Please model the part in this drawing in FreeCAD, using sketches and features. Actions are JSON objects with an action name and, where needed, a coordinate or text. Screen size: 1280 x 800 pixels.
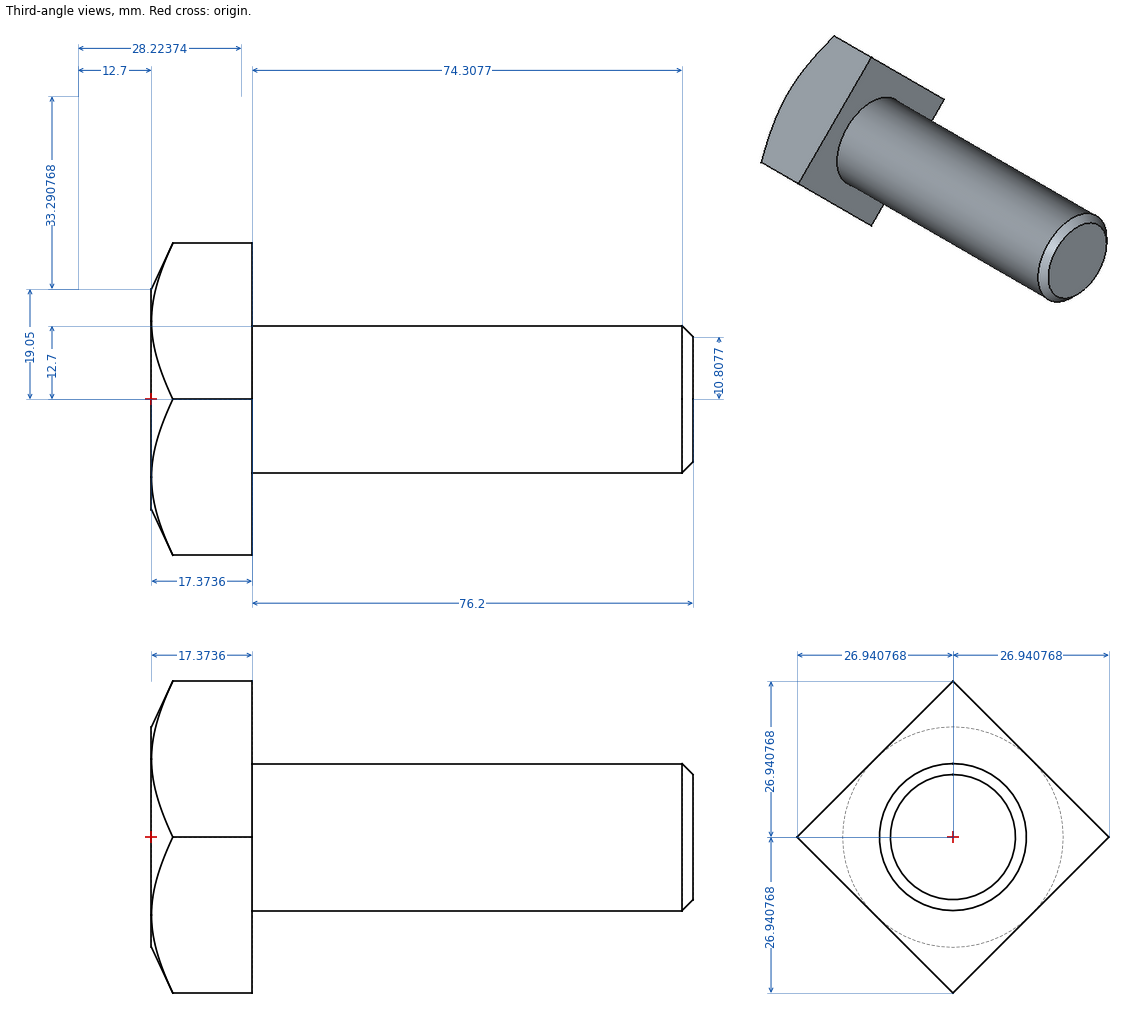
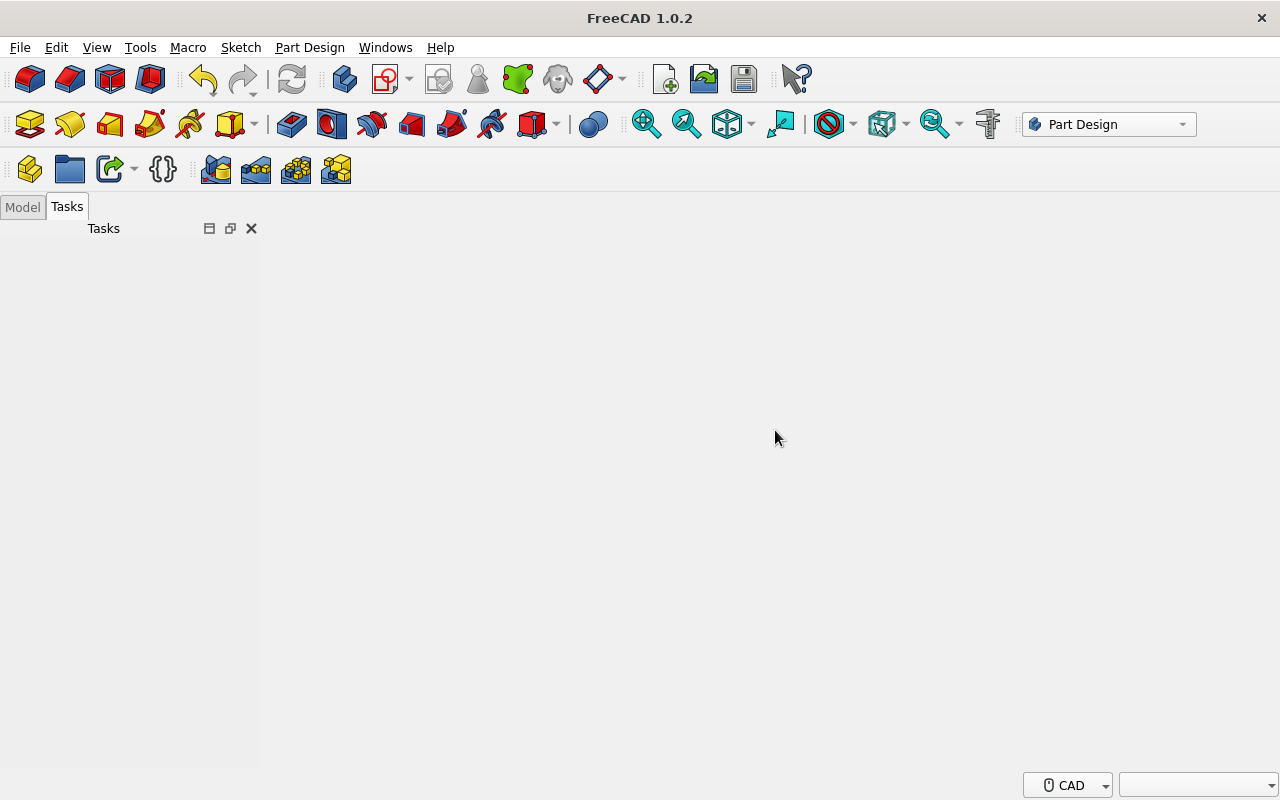
{"action": "left_click", "coordinate": [664, 80]}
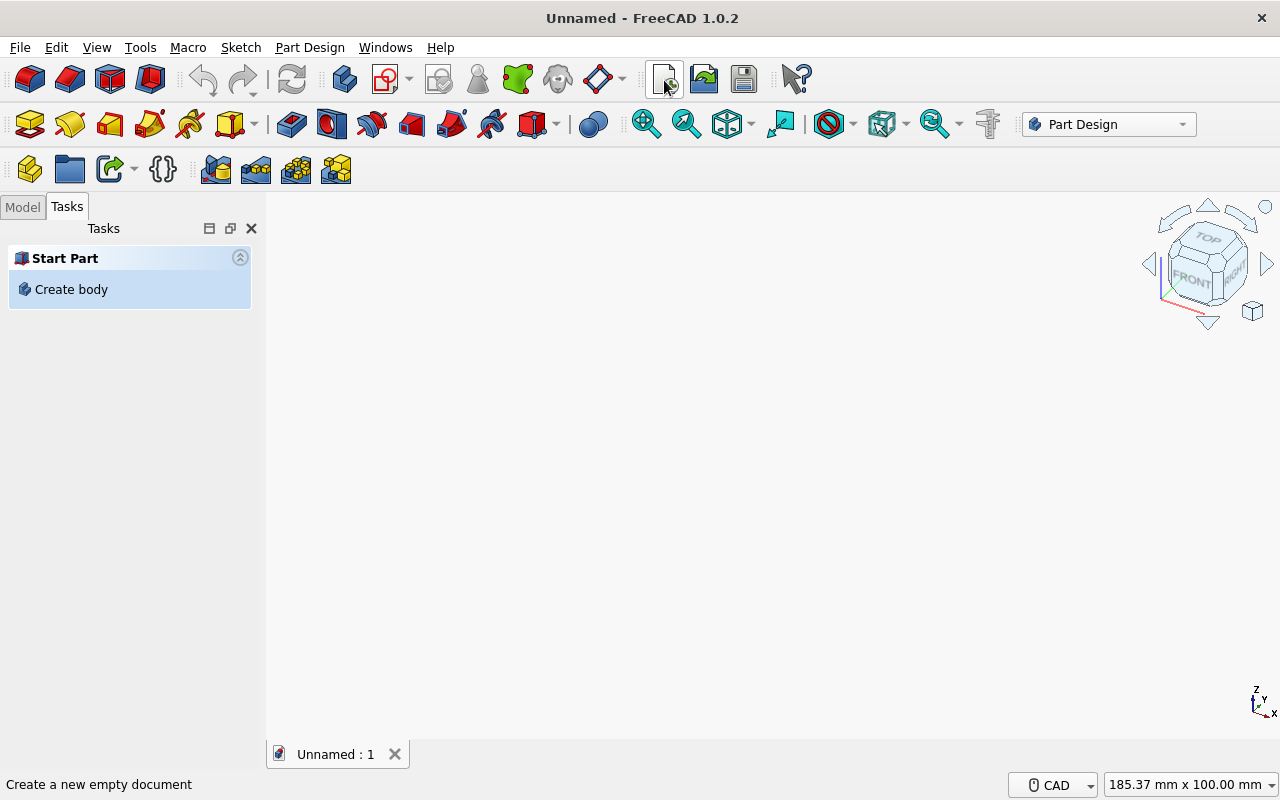
{"action": "left_click", "coordinate": [386, 80]}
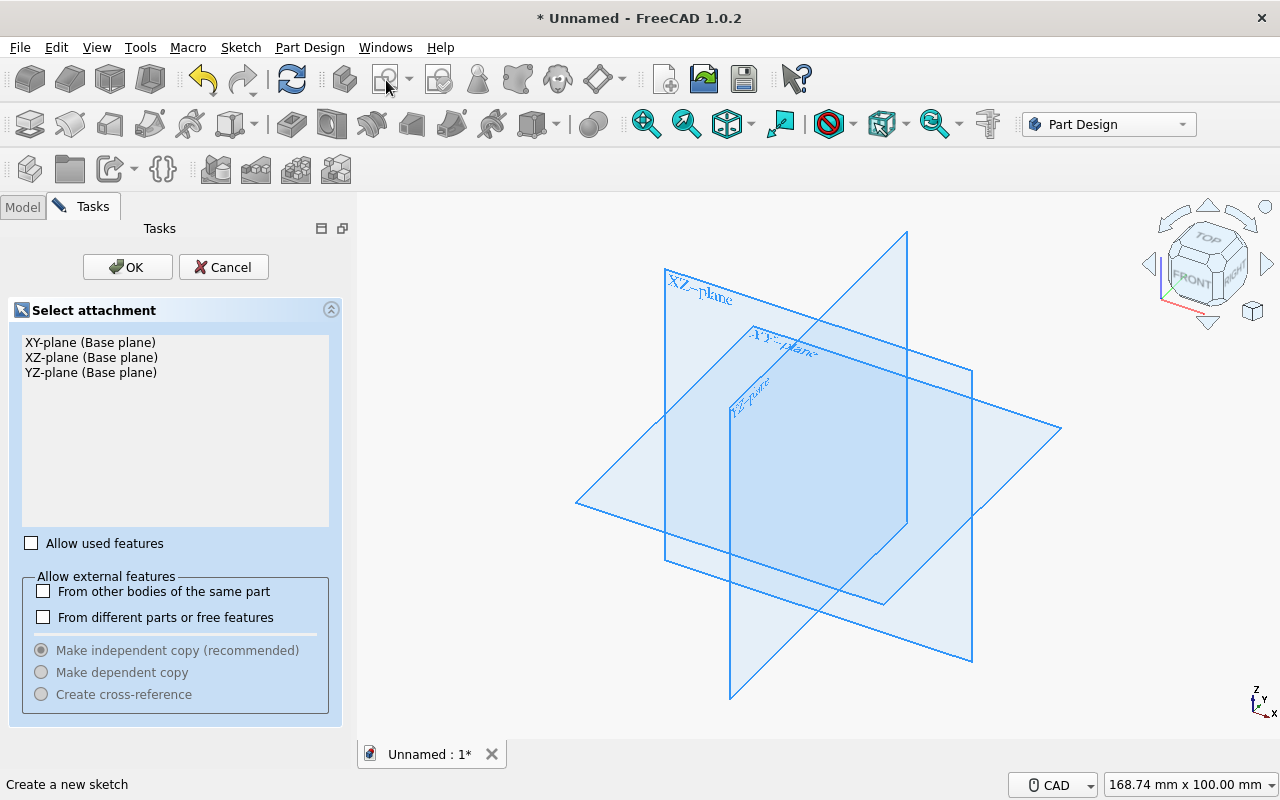
{"action": "left_click", "coordinate": [82, 372]}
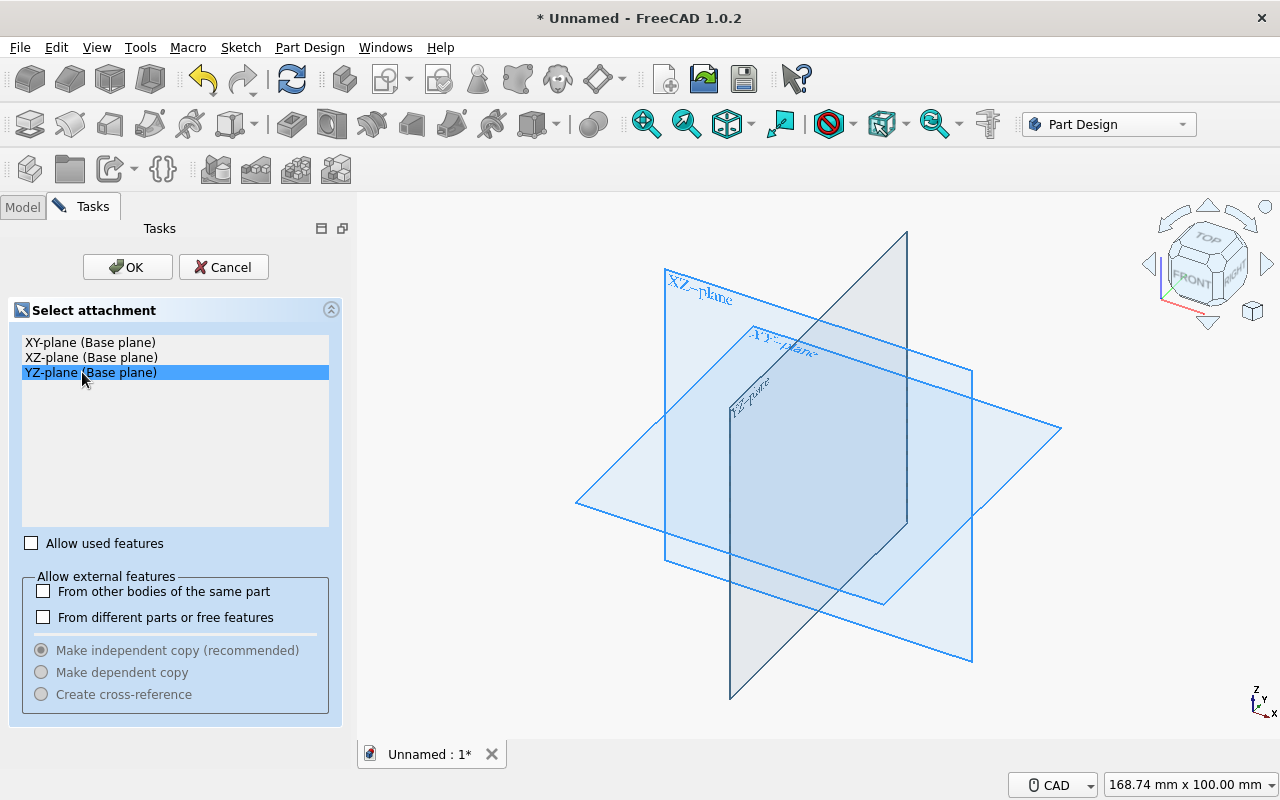
{"action": "left_click", "coordinate": [128, 267]}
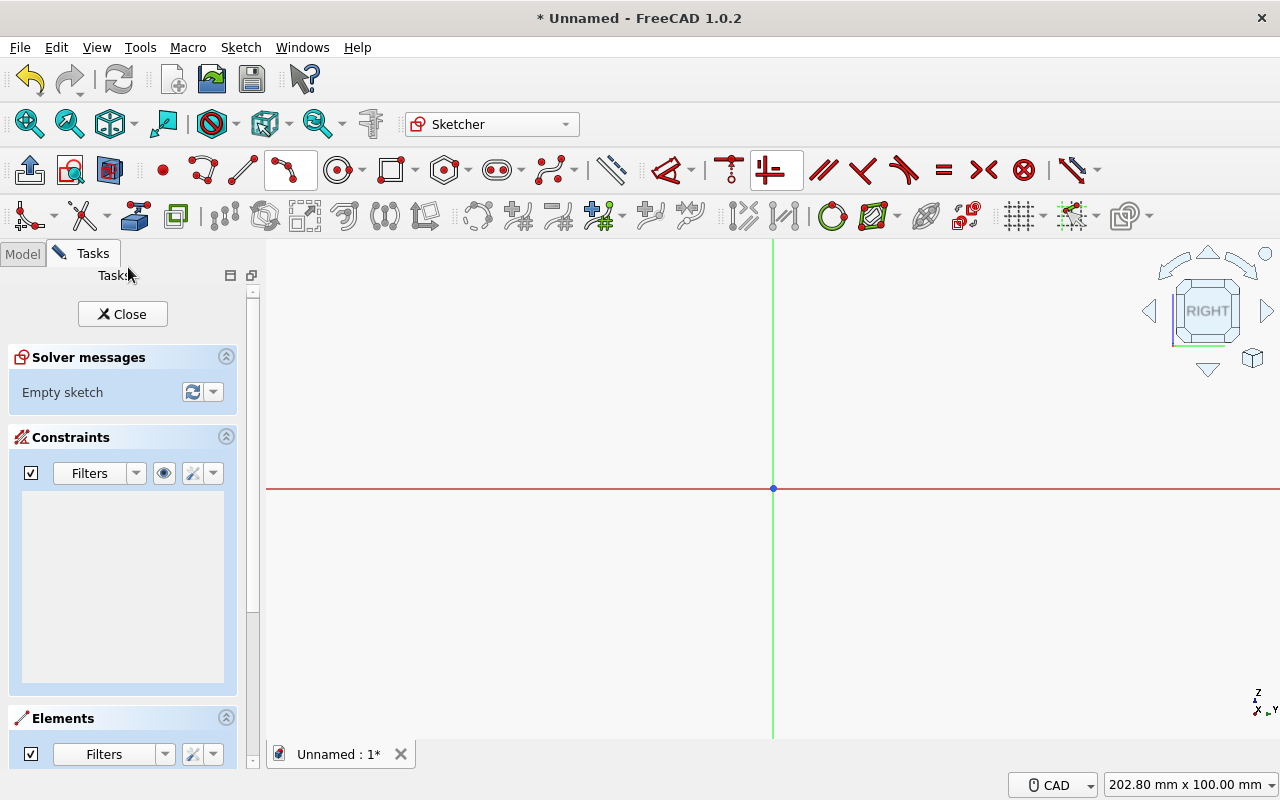
{"action": "left_click", "coordinate": [204, 170]}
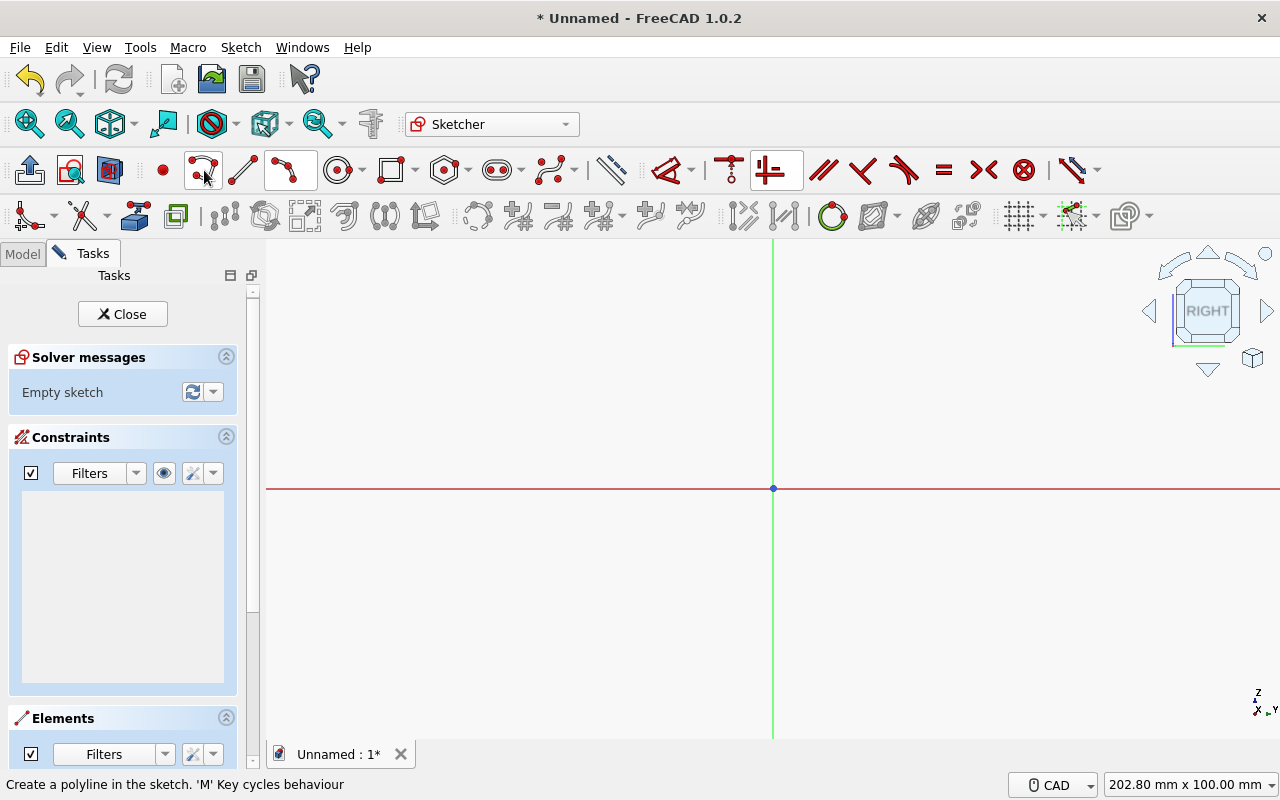
{"action": "left_click", "coordinate": [773, 354]}
{"action": "left_click", "coordinate": [638, 489]}
{"action": "left_click", "coordinate": [773, 624]}
{"action": "left_click", "coordinate": [908, 489]}
{"action": "left_click", "coordinate": [773, 355]}
{"action": "key", "text": "Escape"}
{"action": "key", "text": "Escape"}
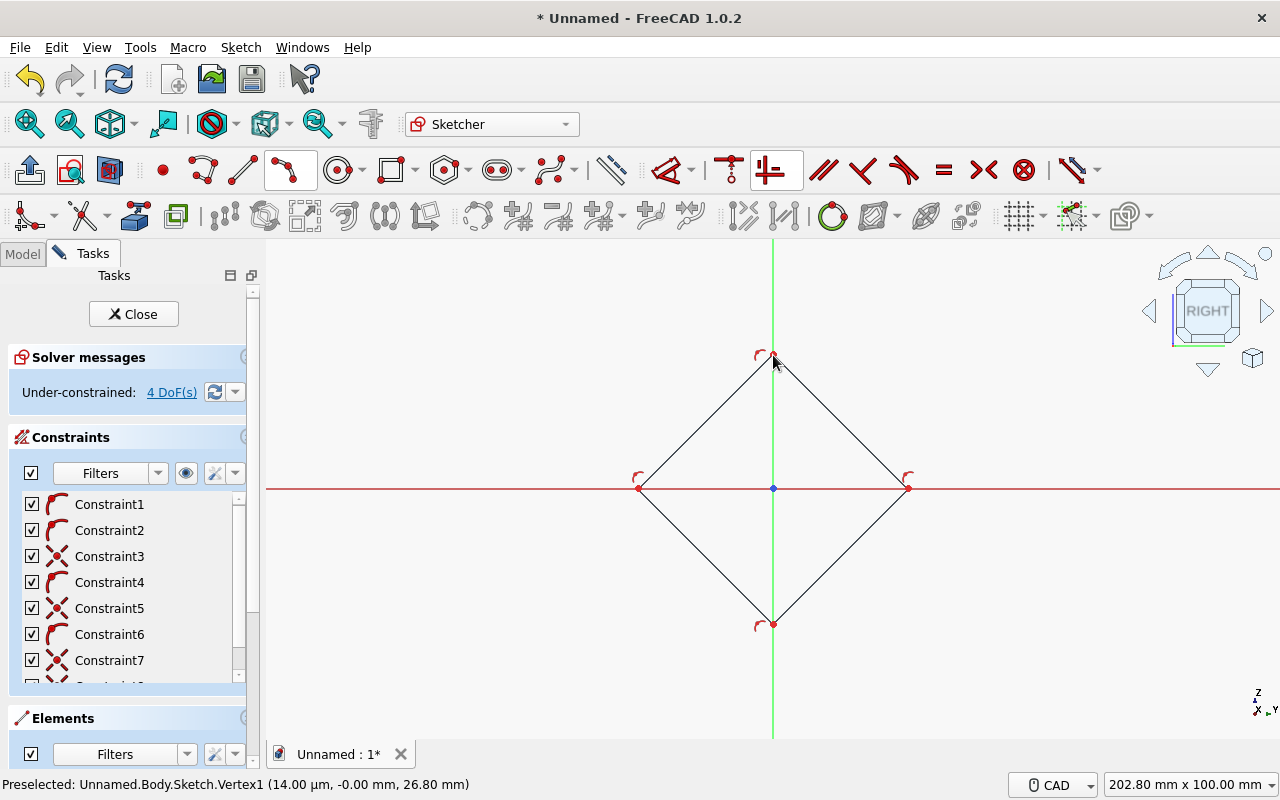
{"action": "left_click", "coordinate": [666, 170]}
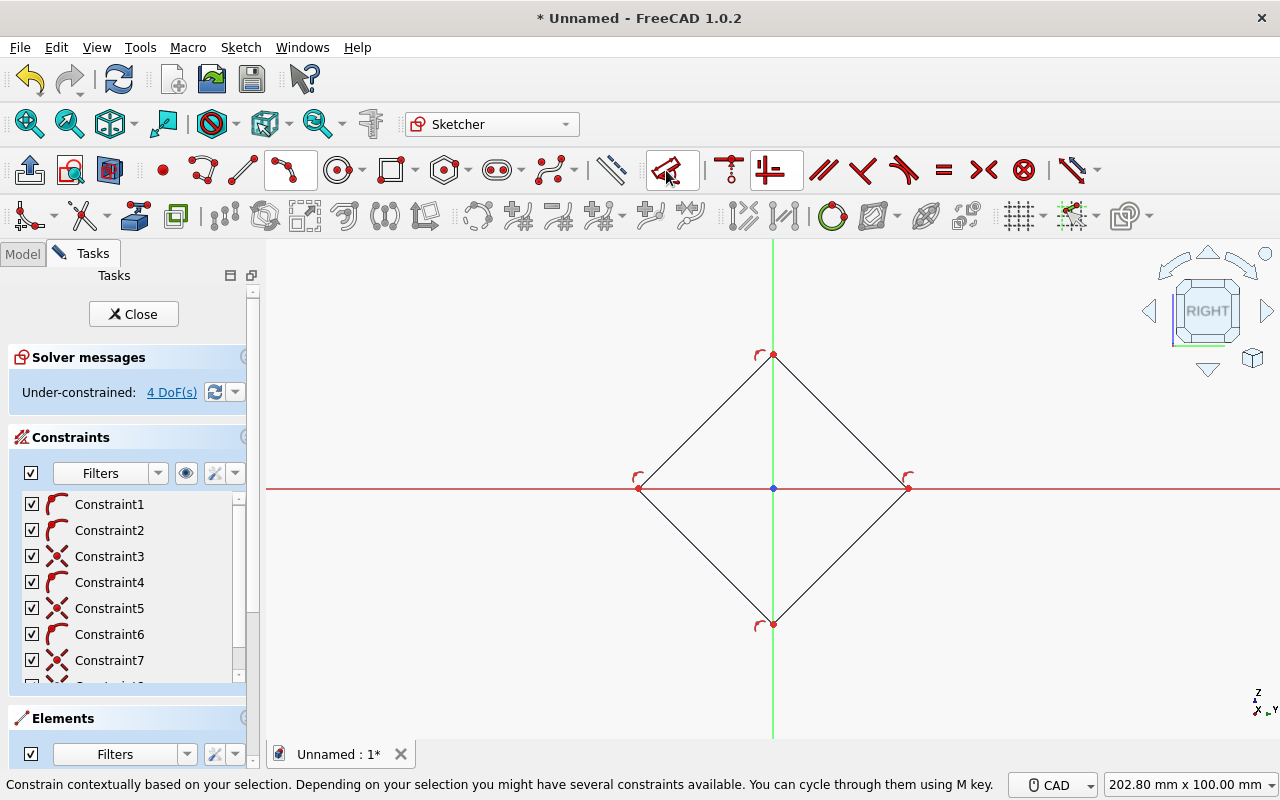
{"action": "left_click", "coordinate": [773, 355]}
{"action": "left_click", "coordinate": [807, 422]}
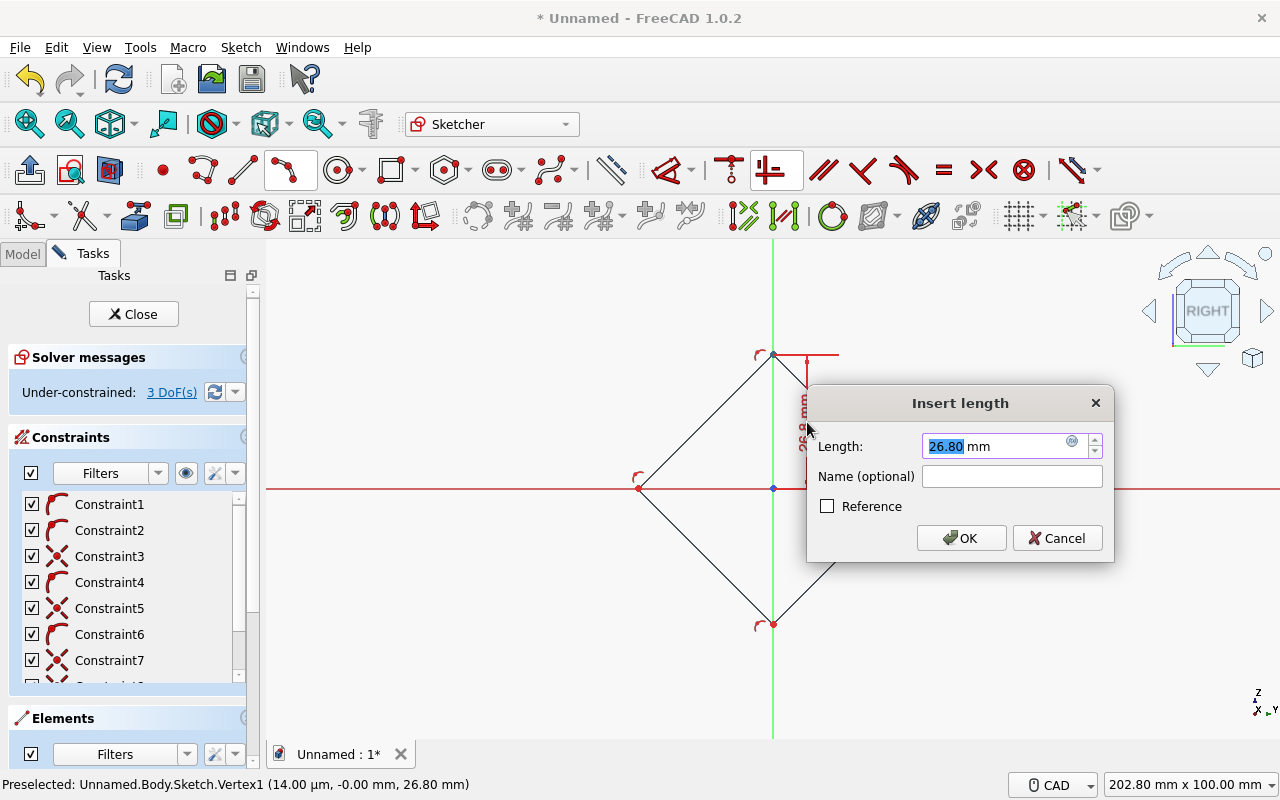
{"action": "type", "text": "26.940768"}
{"action": "key", "text": "Return"}